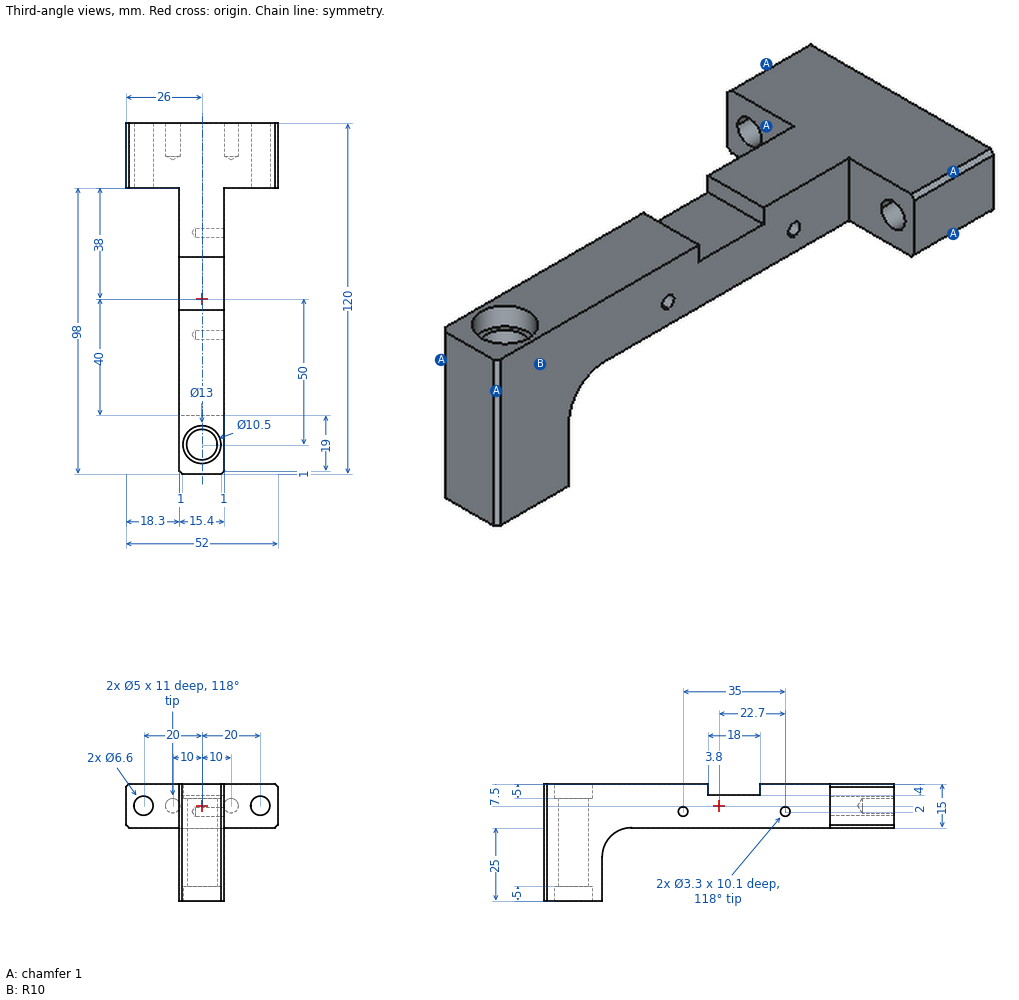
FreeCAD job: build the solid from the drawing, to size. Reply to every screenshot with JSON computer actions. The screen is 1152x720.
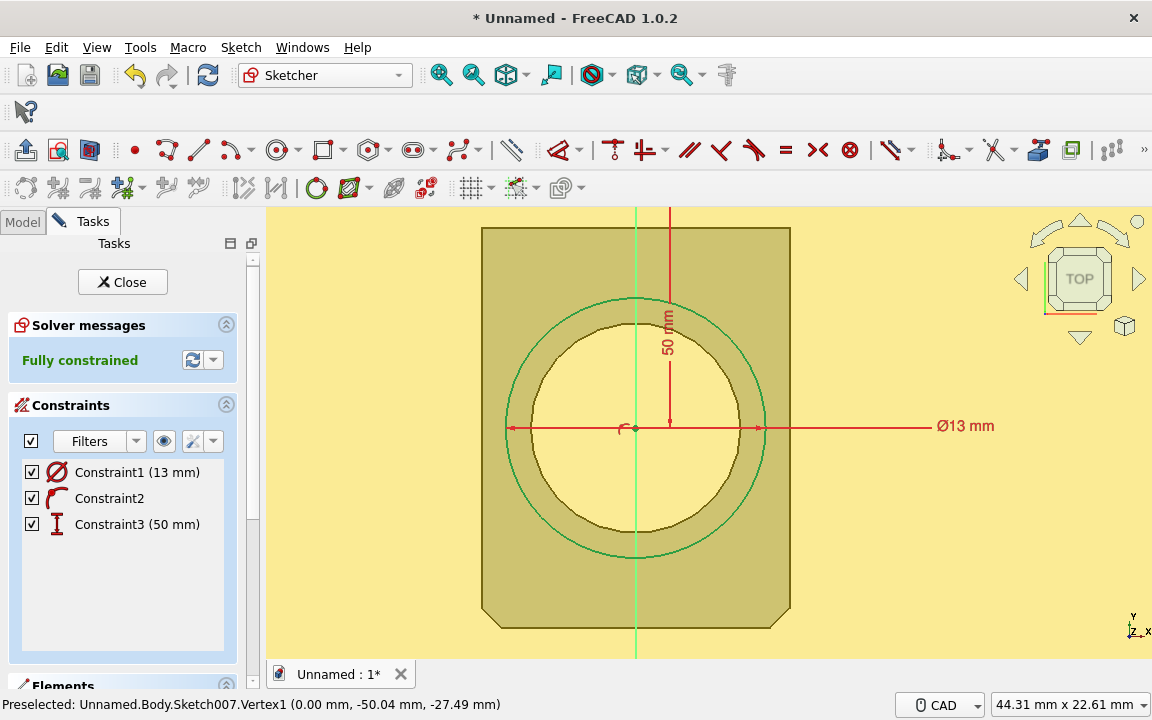
{"action": "left_click", "coordinate": [123, 282]}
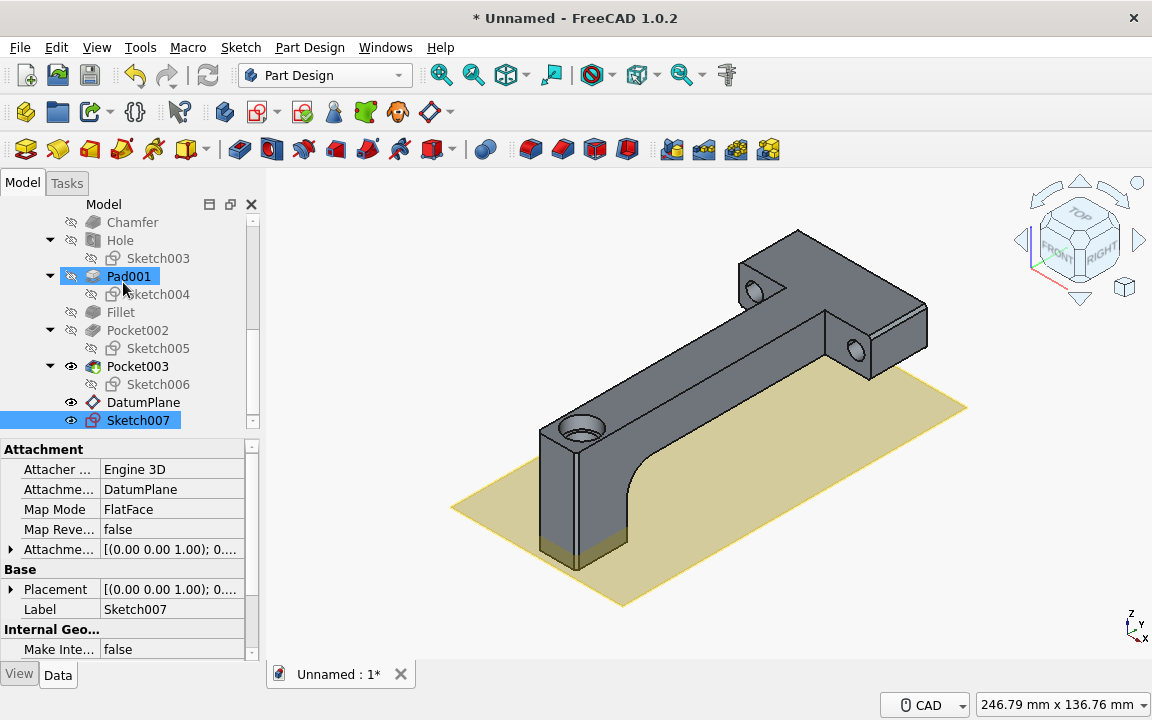
{"action": "left_click", "coordinate": [240, 150]}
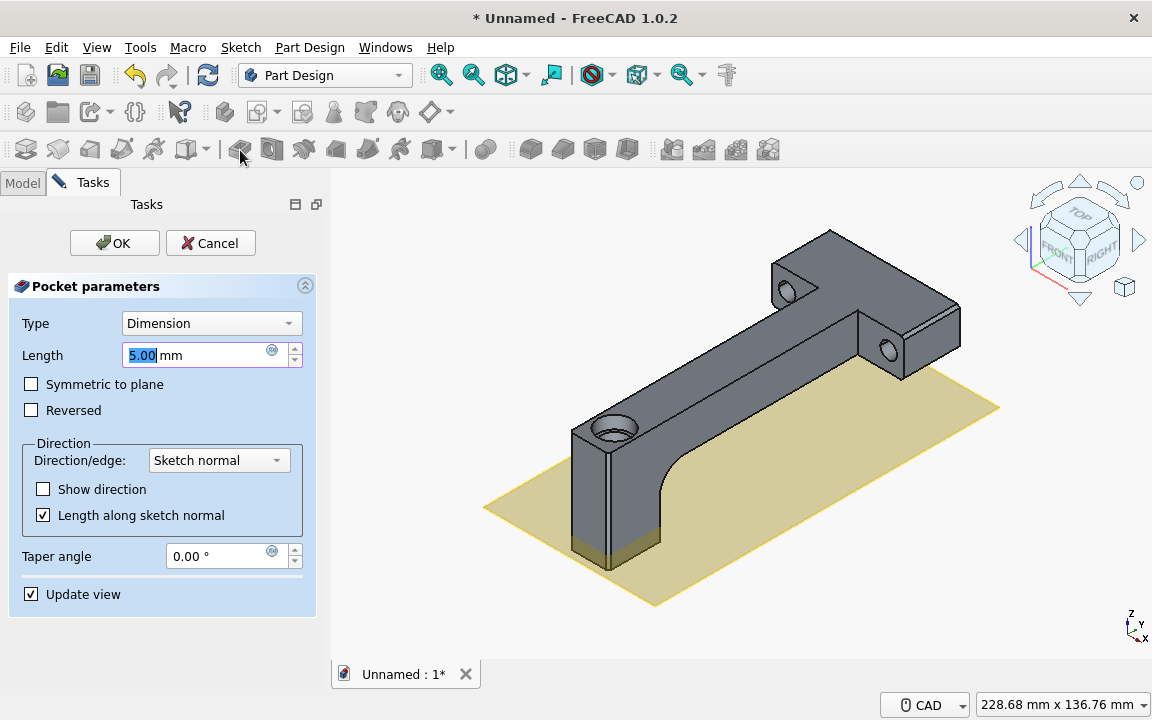
{"action": "type", "text": "5"}
{"action": "key", "text": "Tab"}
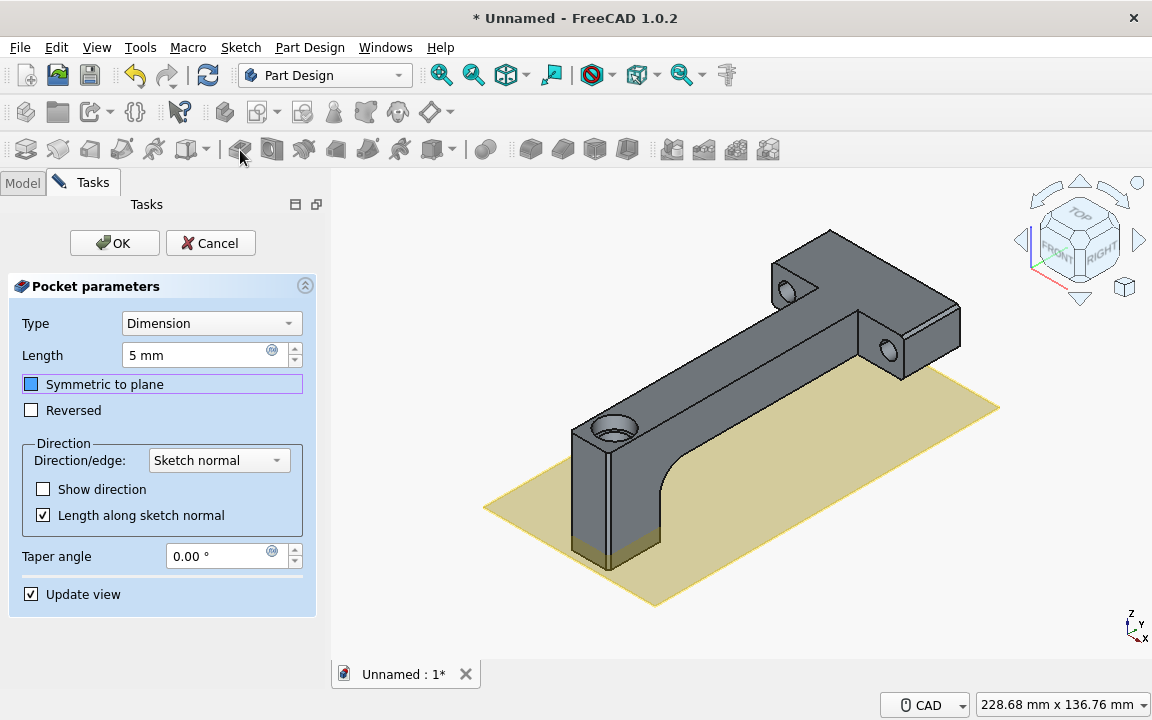
{"action": "left_click", "coordinate": [115, 243]}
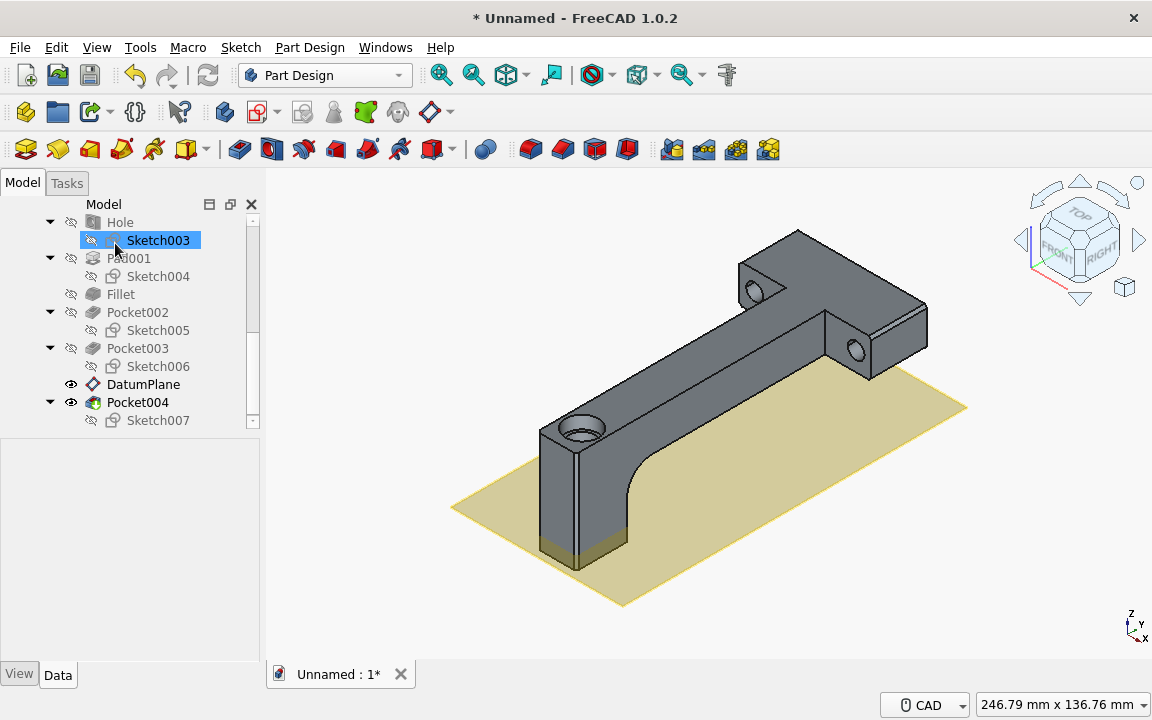
{"action": "left_click", "coordinate": [116, 384]}
{"action": "key", "text": "space"}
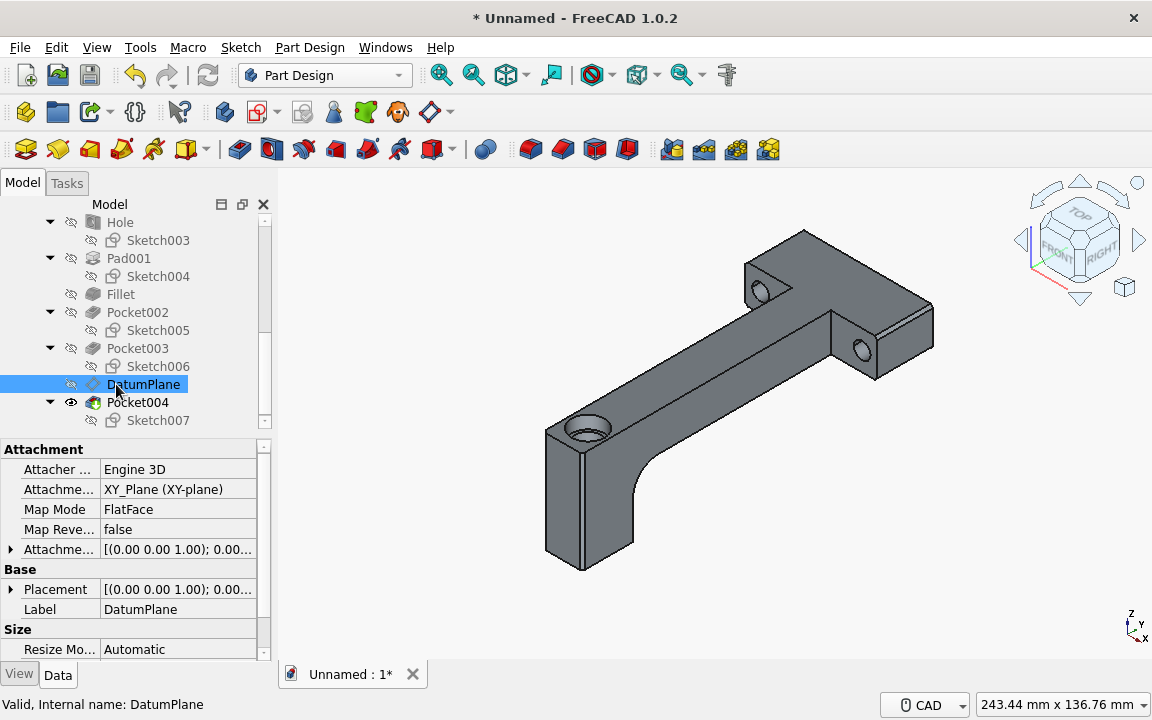
{"action": "left_click", "coordinate": [638, 446]}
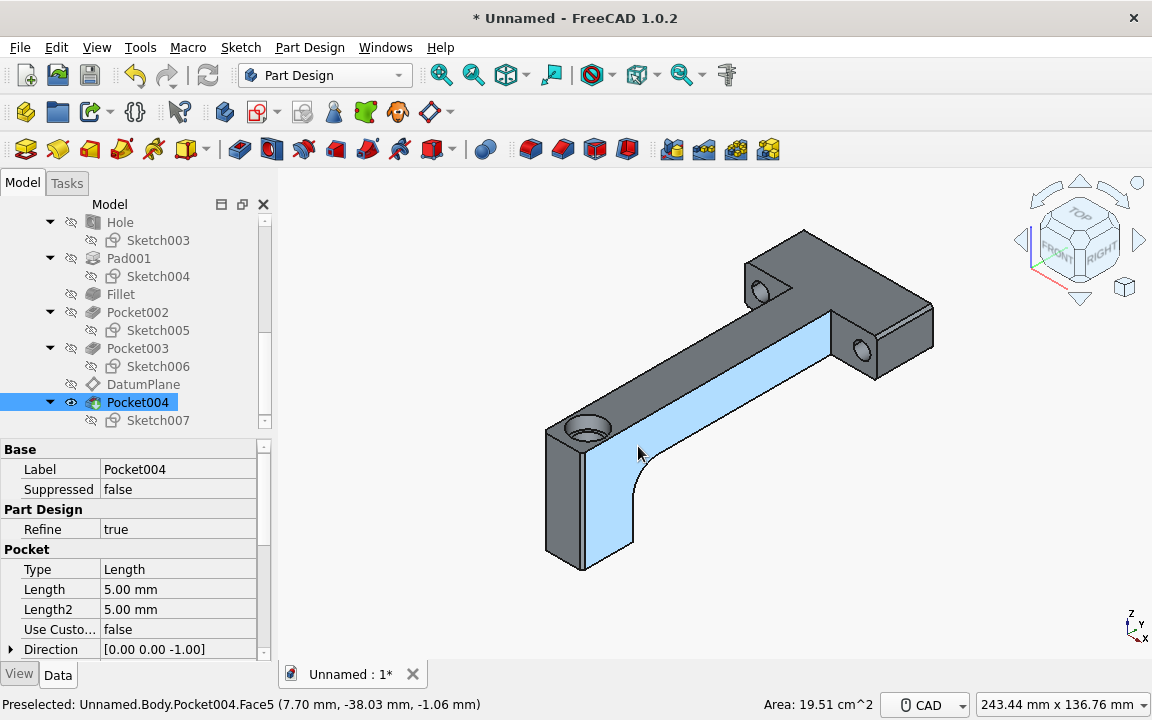
{"action": "left_click", "coordinate": [258, 112]}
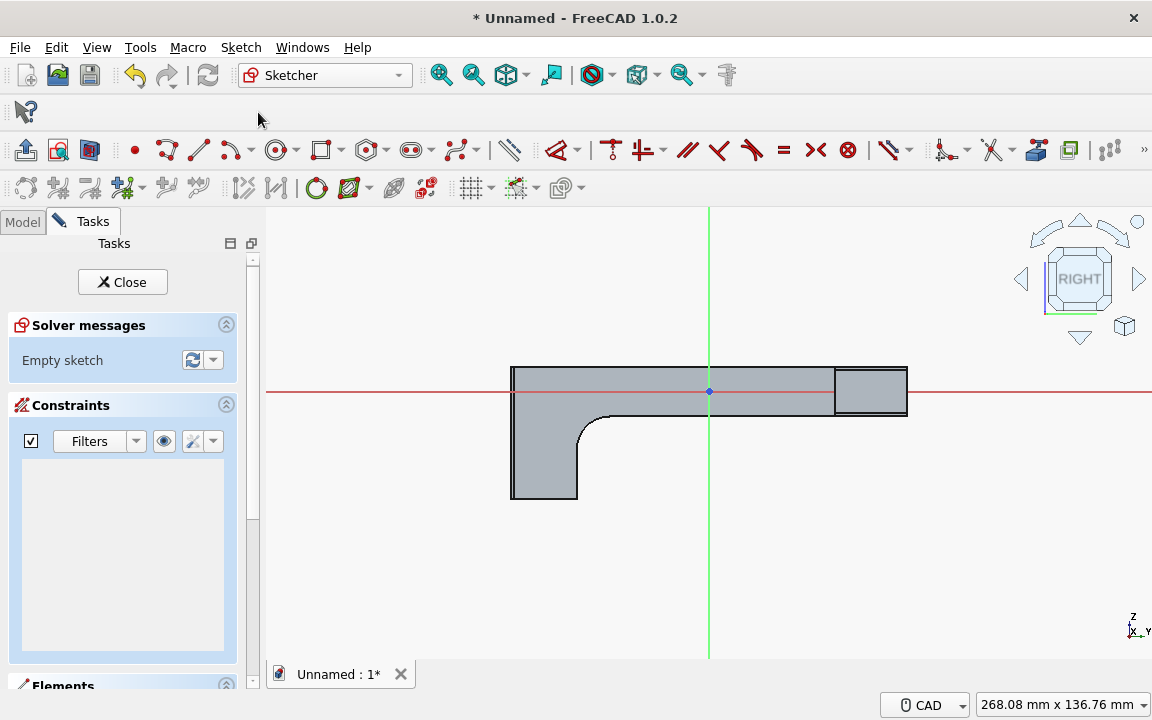
{"action": "scroll", "coordinate": [737, 373], "scroll_direction": "up", "scroll_amount": 11}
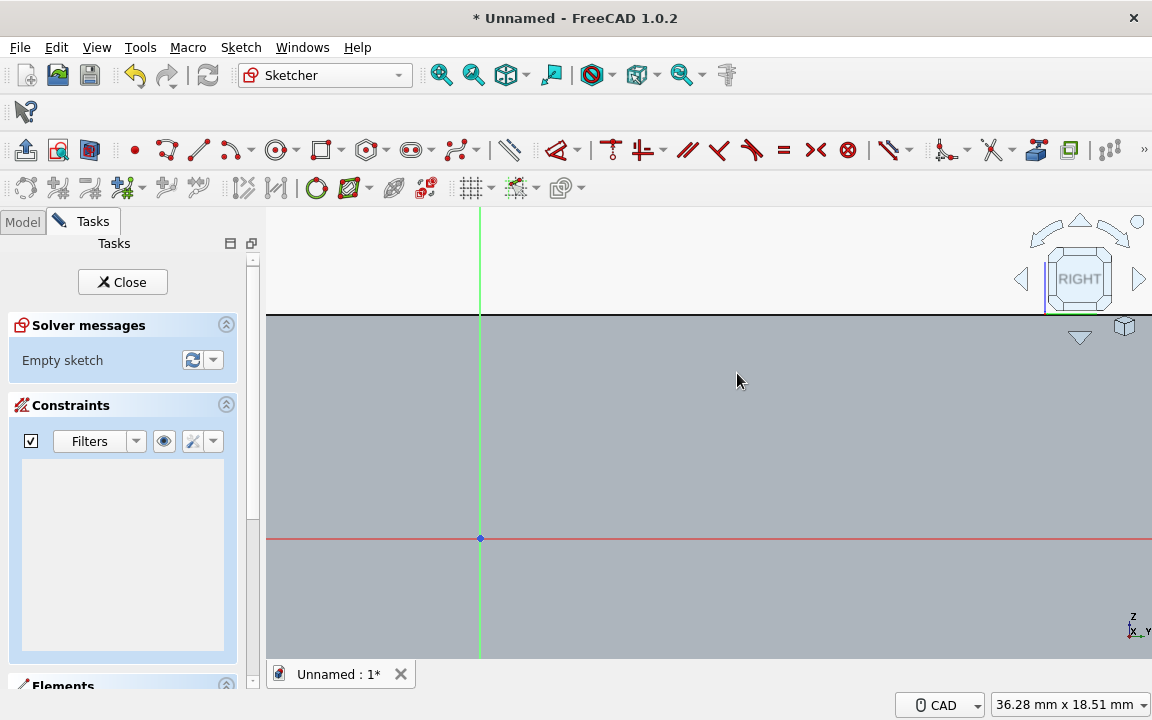
{"action": "left_click", "coordinate": [322, 150]}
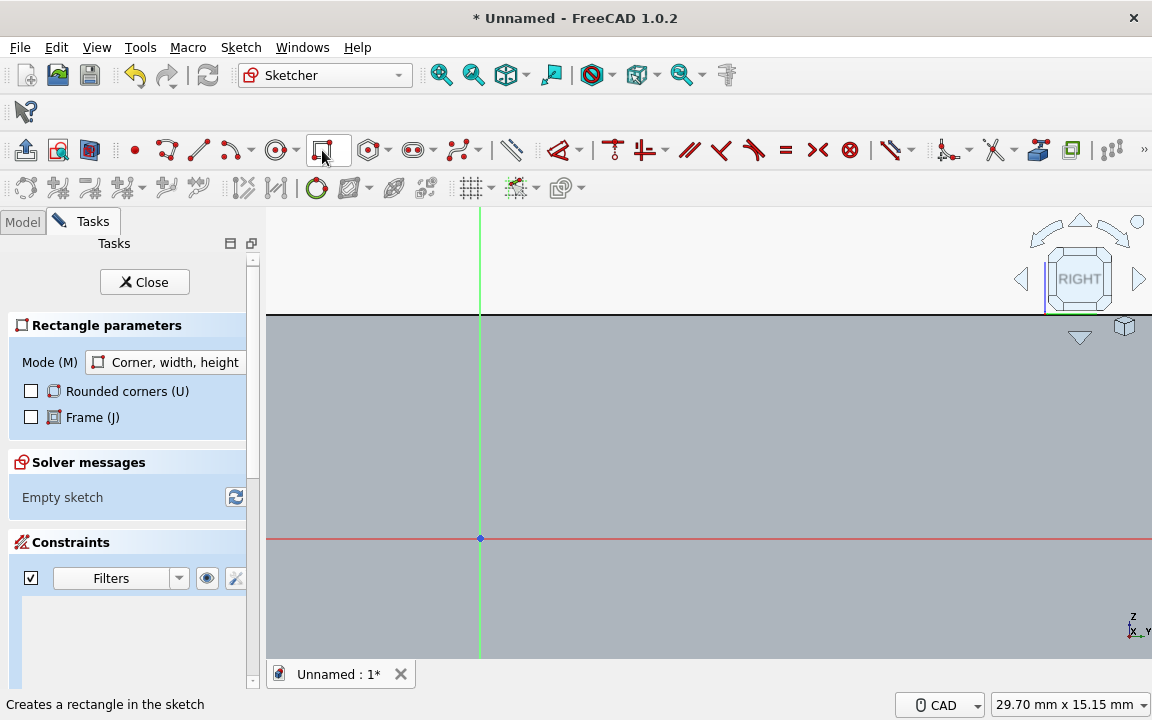
{"action": "left_click", "coordinate": [367, 315]}
{"action": "mouse_move", "coordinate": [904, 434]}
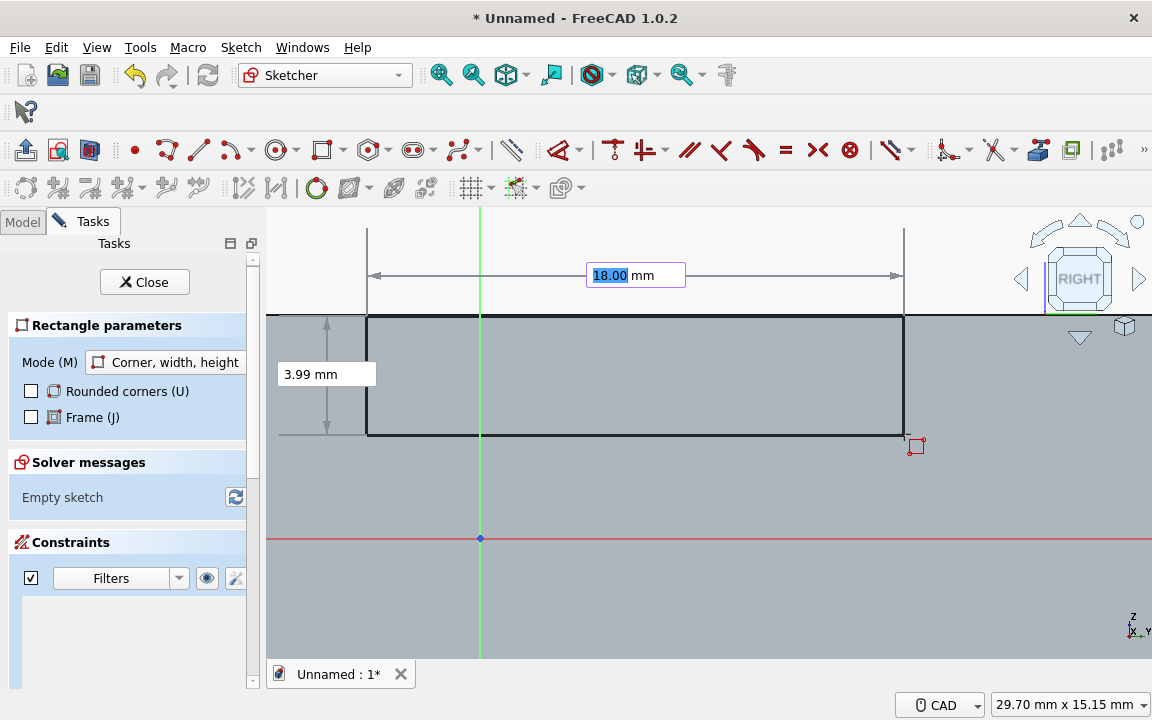
{"action": "type", "text": "18"}
{"action": "key", "text": "Tab"}
{"action": "type", "text": "4"}
{"action": "key", "text": "Return"}
{"action": "key", "text": "Escape"}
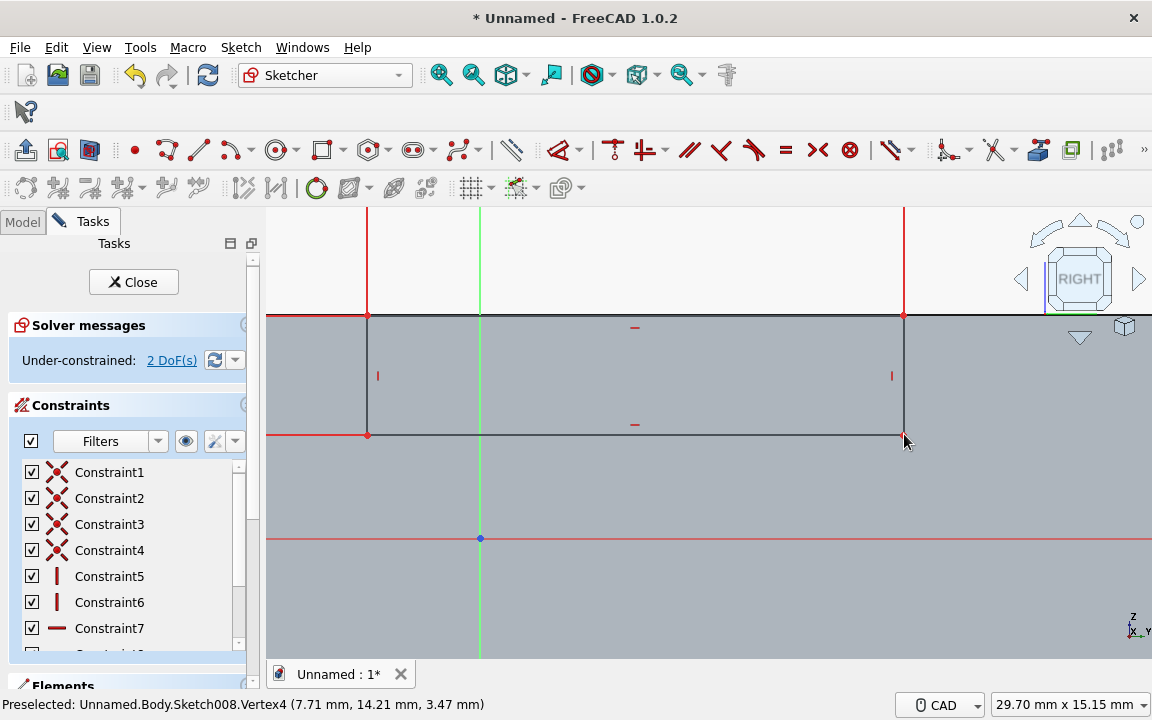
{"action": "left_click", "coordinate": [558, 150]}